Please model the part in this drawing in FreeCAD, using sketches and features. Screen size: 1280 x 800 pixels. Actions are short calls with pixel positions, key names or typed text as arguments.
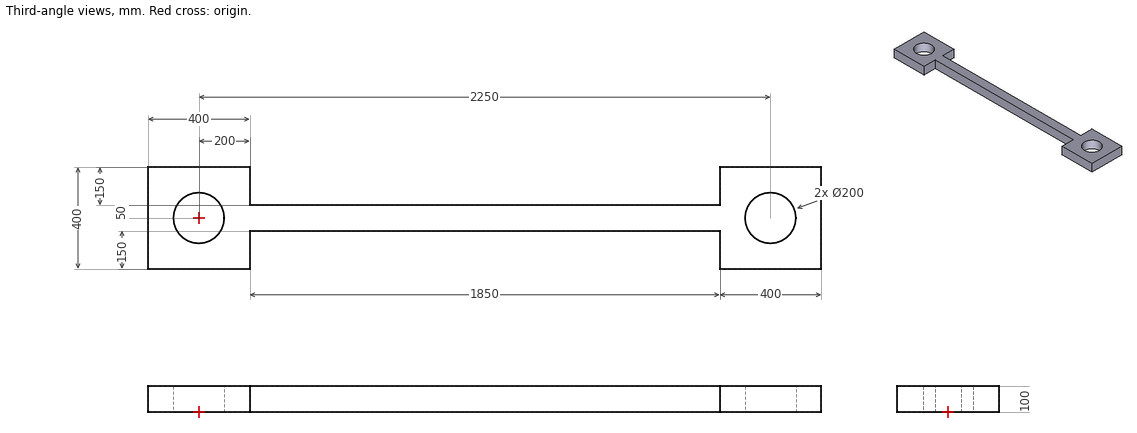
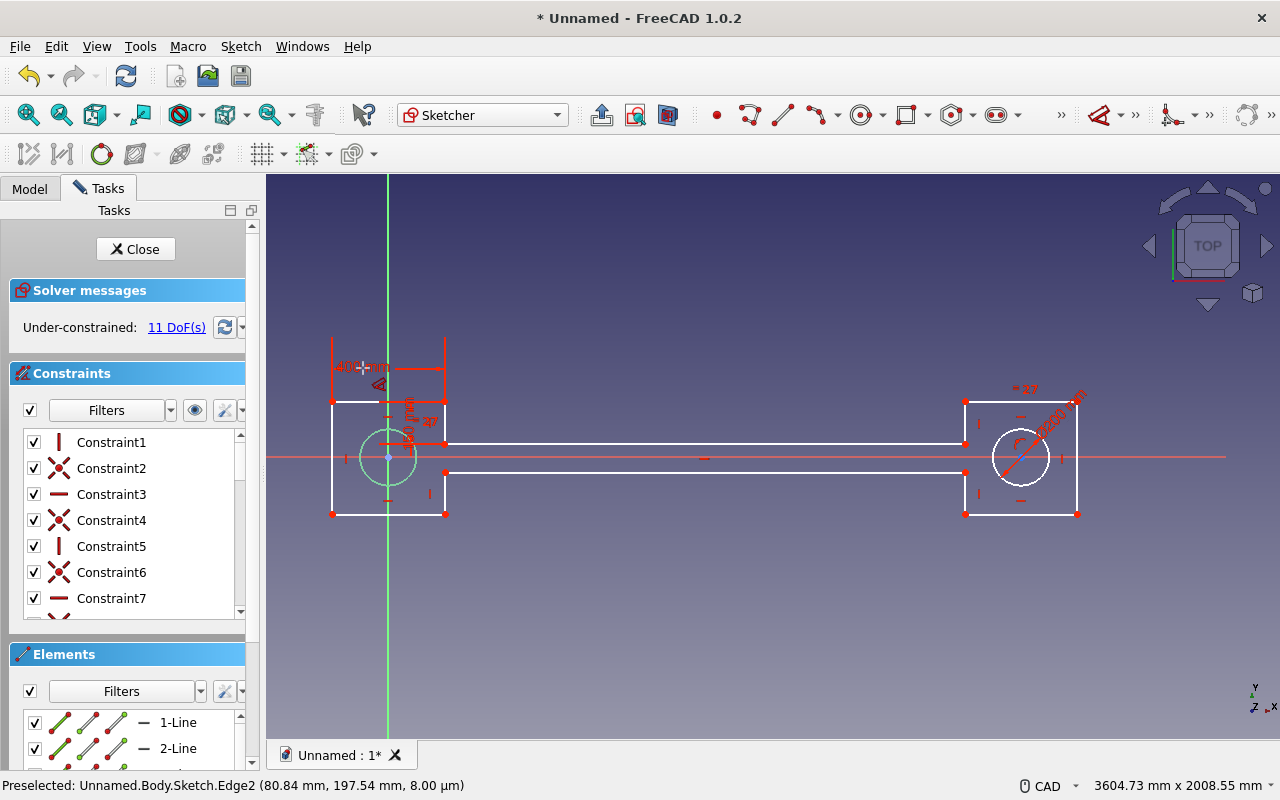
click(332, 436)
click(298, 432)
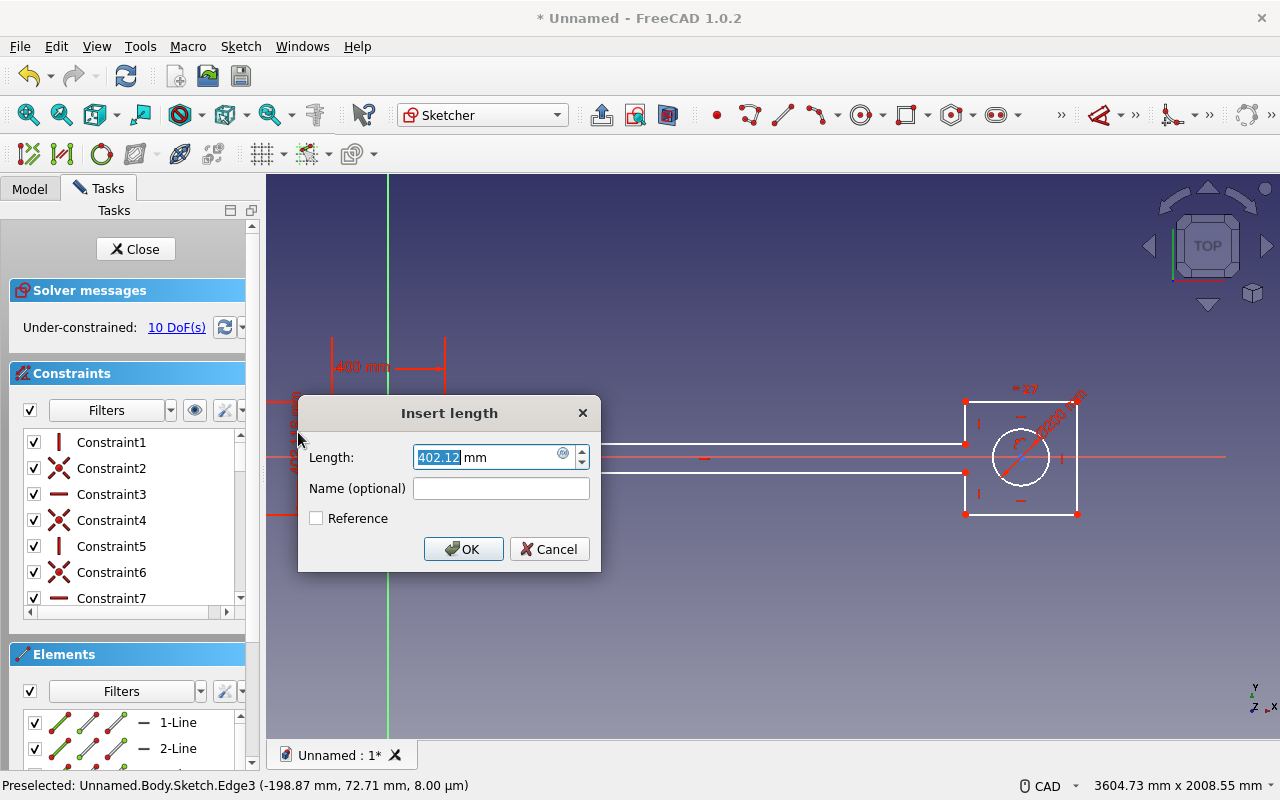
text(400)
key(Return)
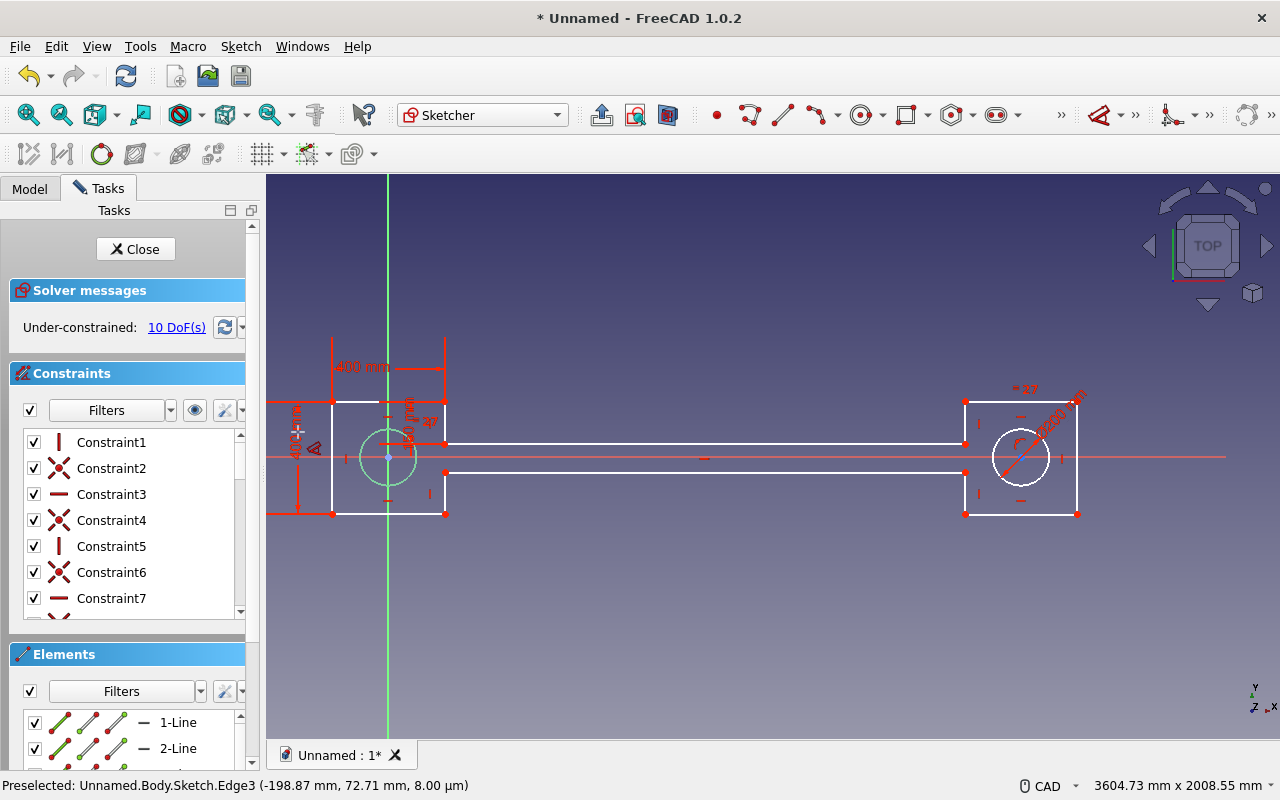
click(366, 514)
click(363, 548)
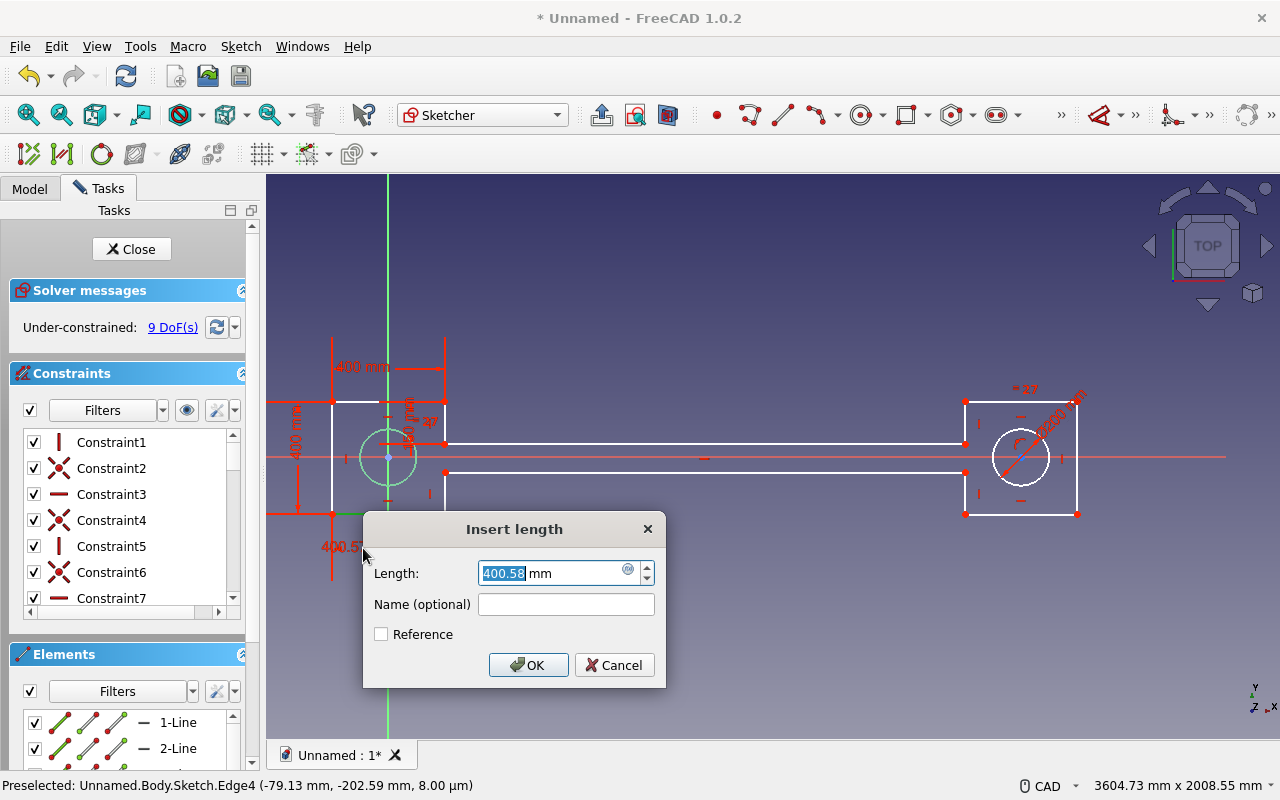
text(400)
key(Return)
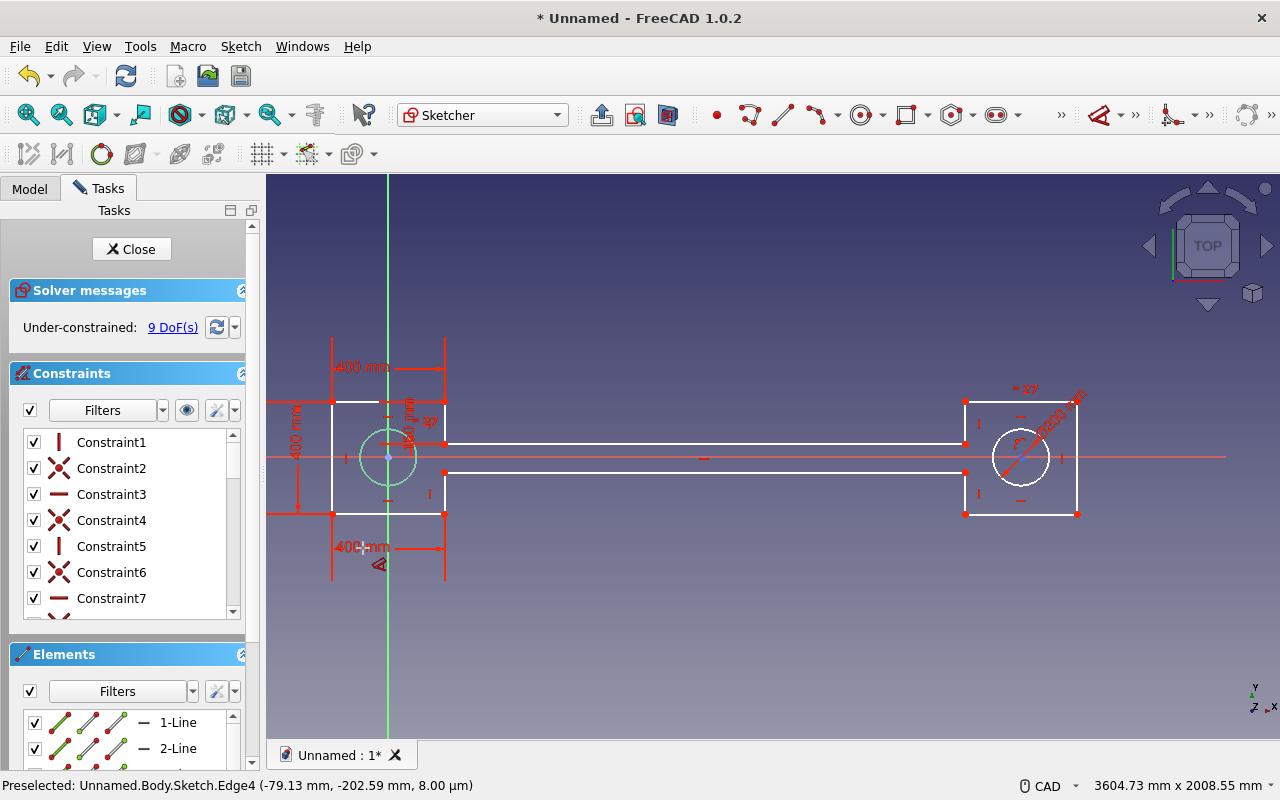
click(445, 502)
click(411, 494)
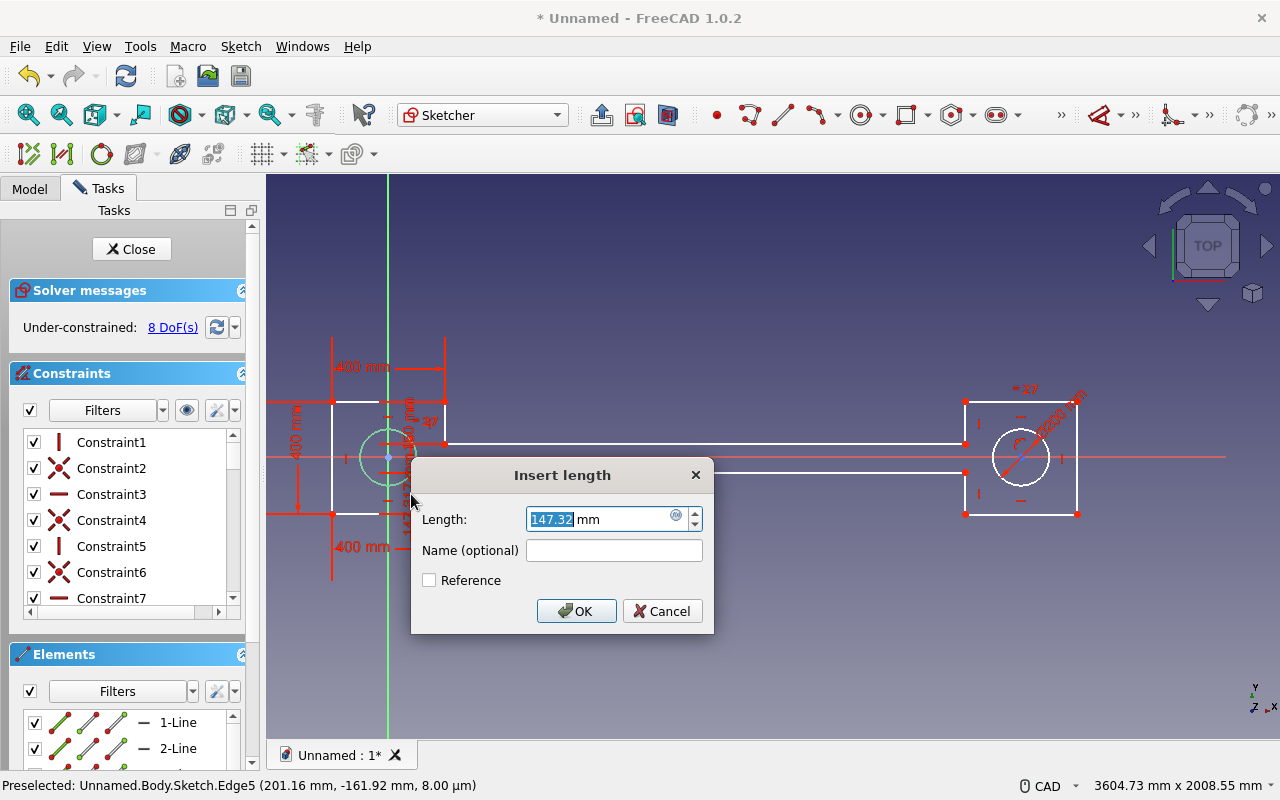
text(150)
key(Return)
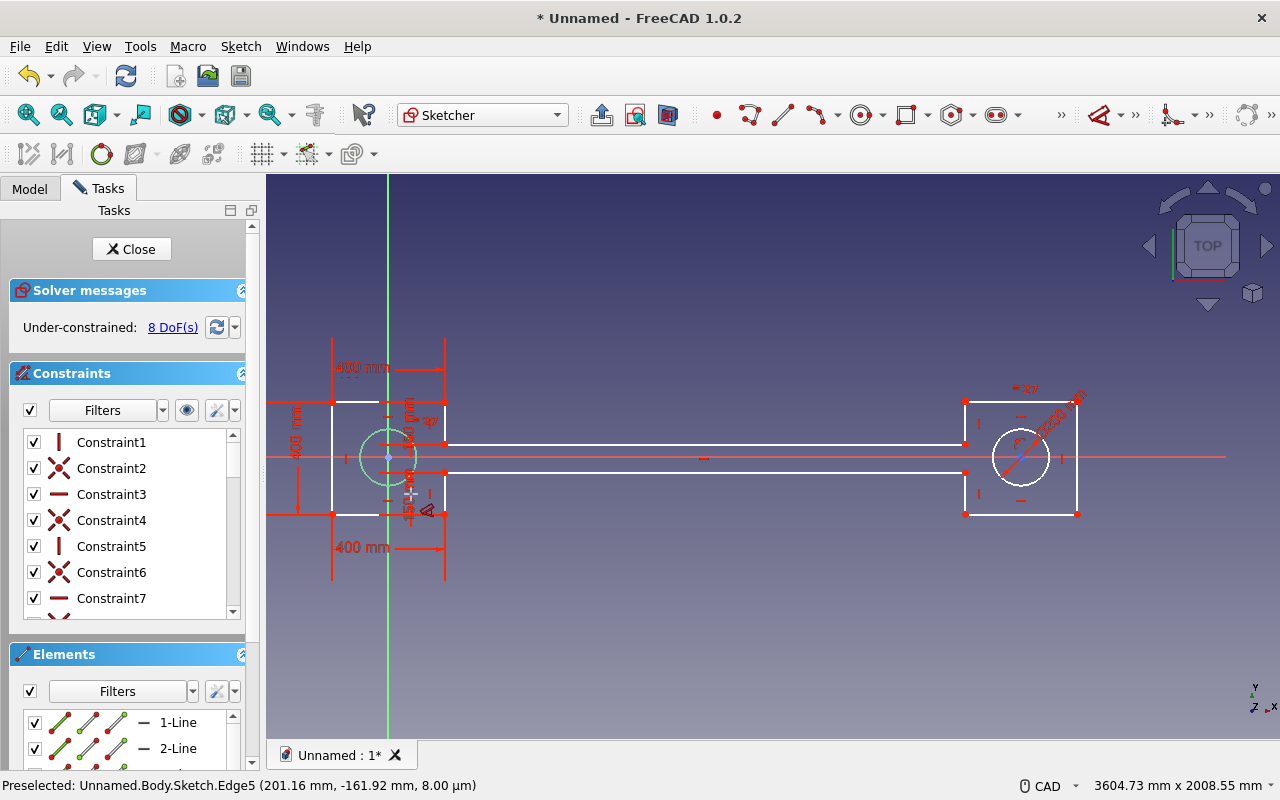
click(965, 485)
click(999, 494)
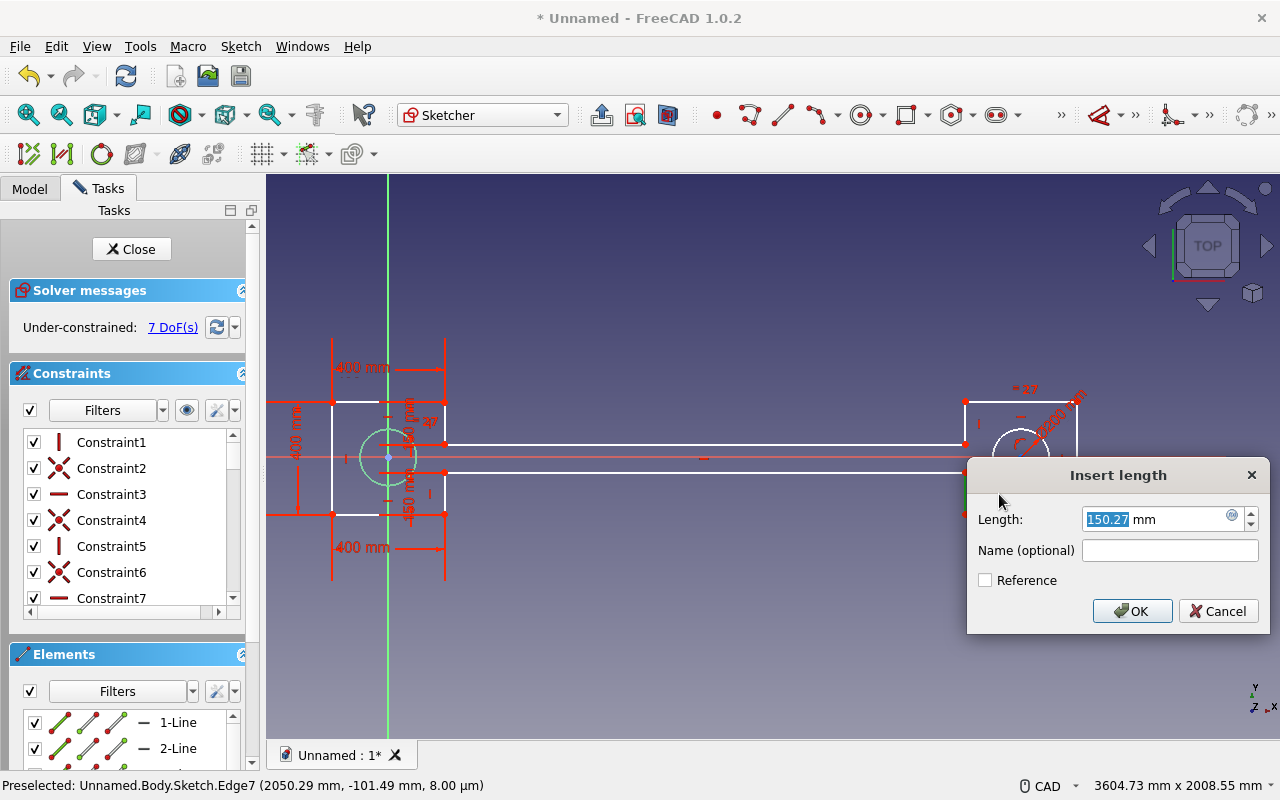
text(150)
key(Return)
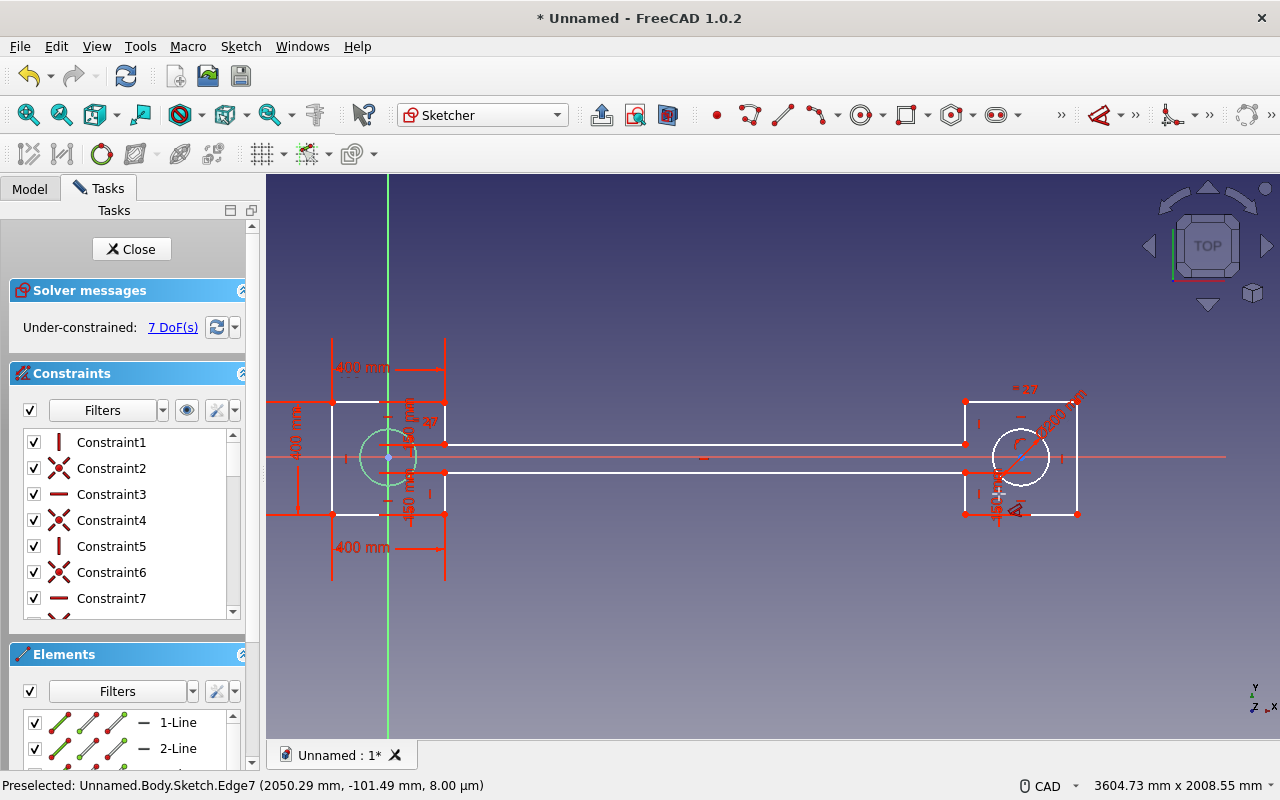
click(999, 515)
click(1021, 549)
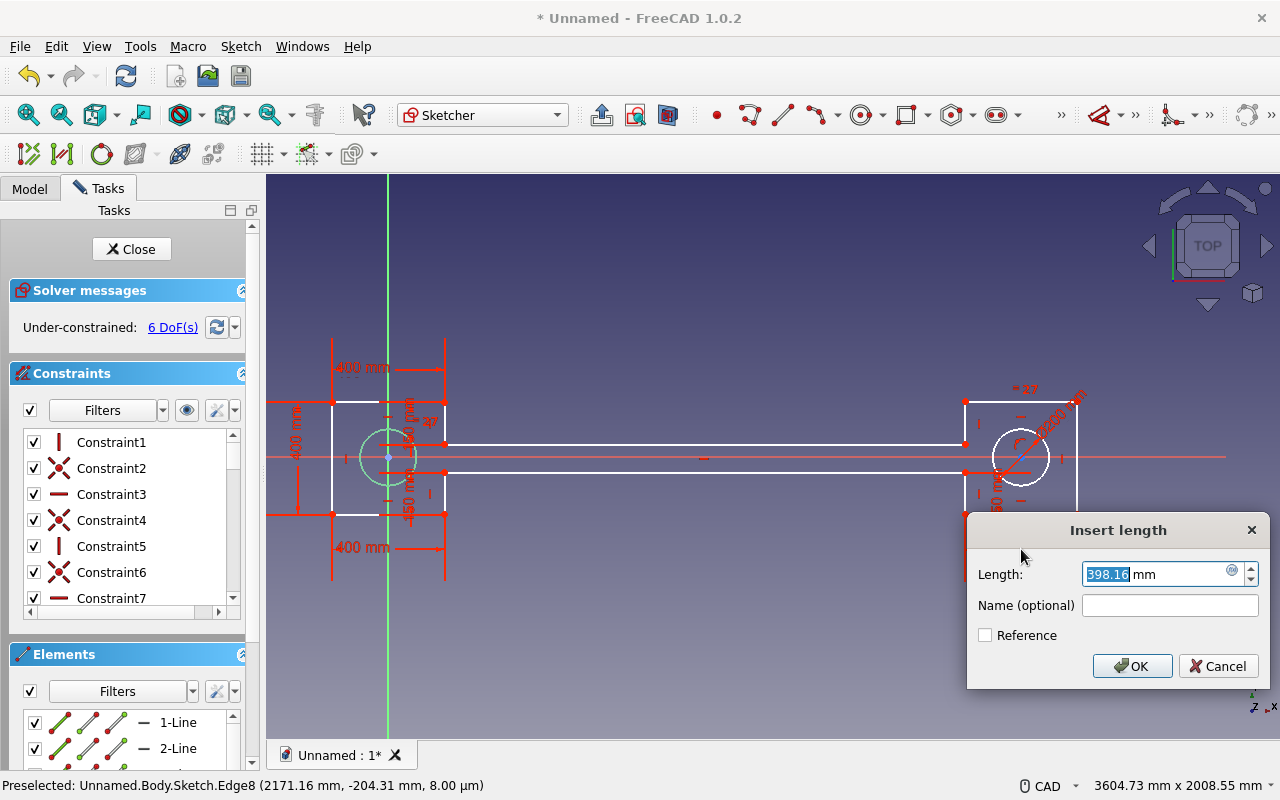
text(400)
key(Return)